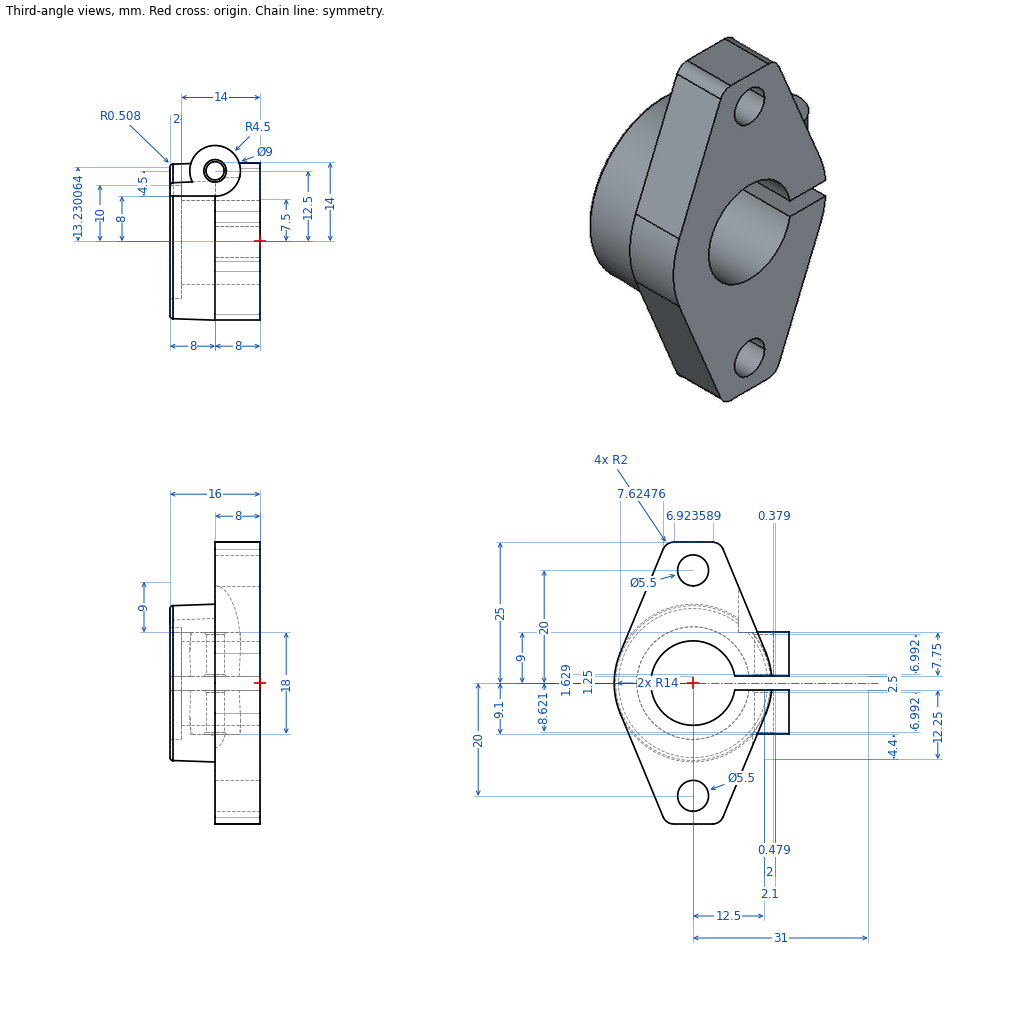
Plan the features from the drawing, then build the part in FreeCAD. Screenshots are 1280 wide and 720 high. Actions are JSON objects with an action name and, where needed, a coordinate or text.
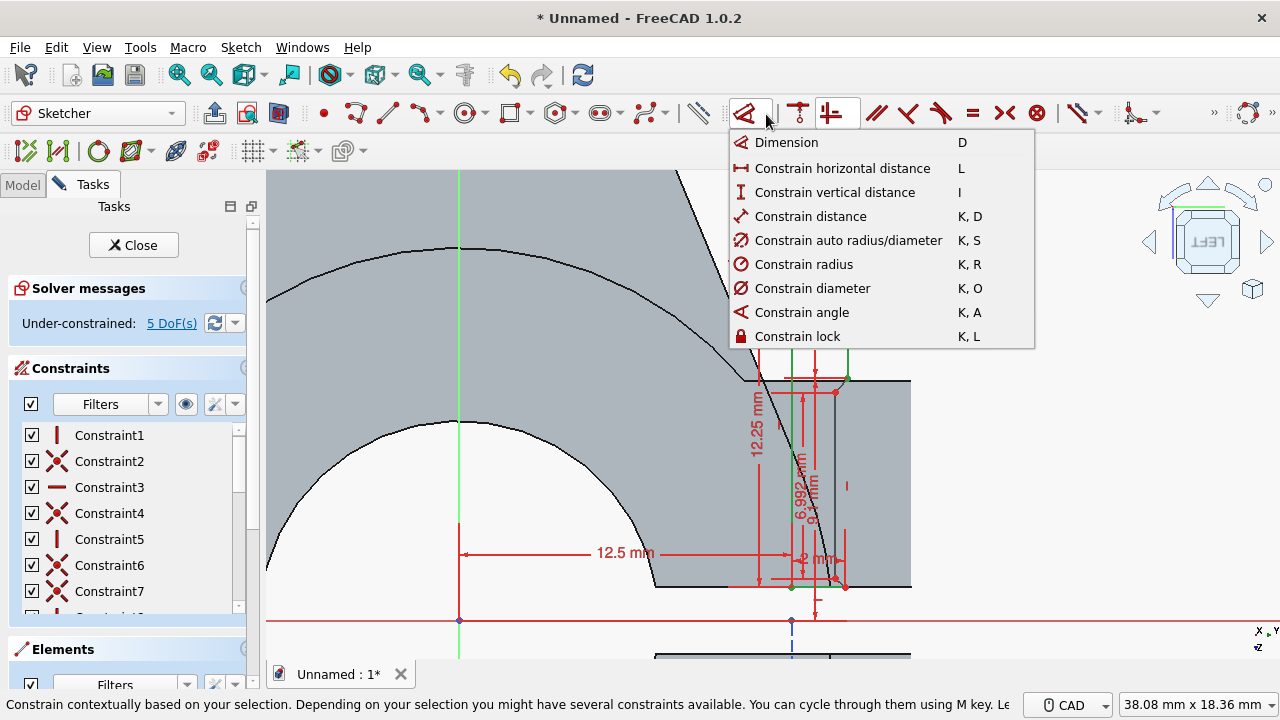
{"action": "left_click", "coordinate": [882, 168]}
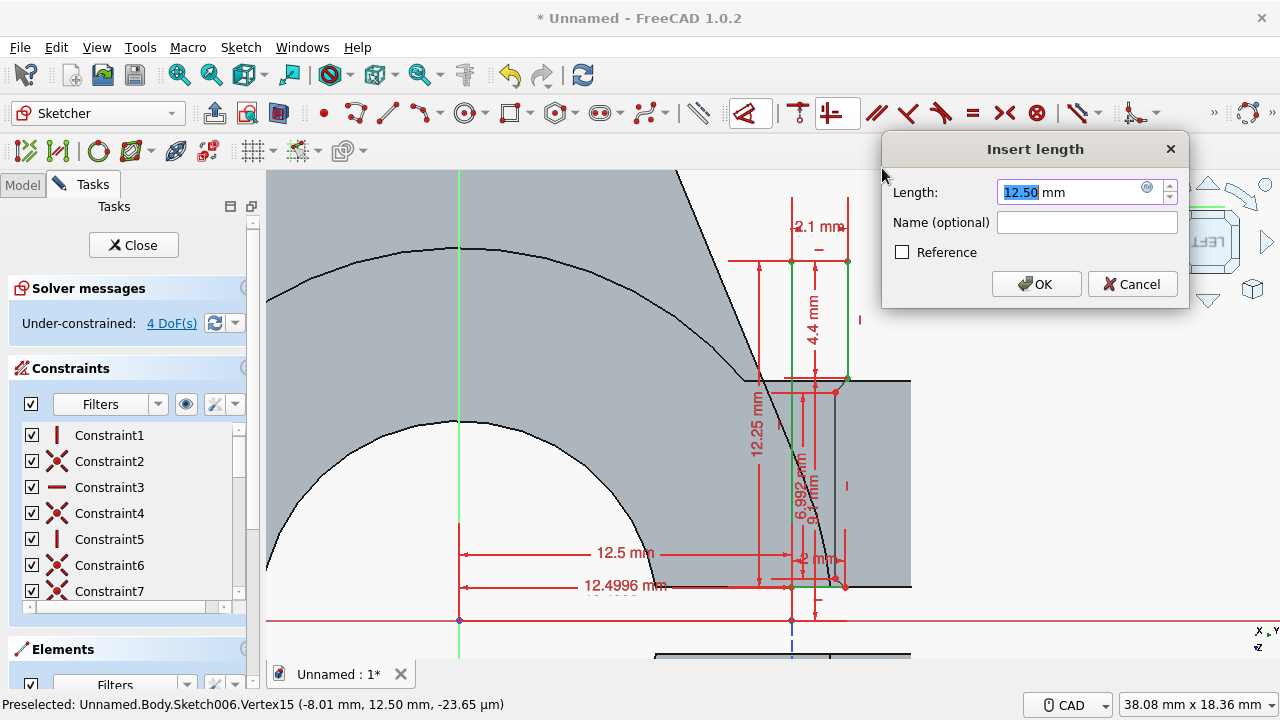
{"action": "type", "text": "12.5"}
{"action": "key", "text": "Return"}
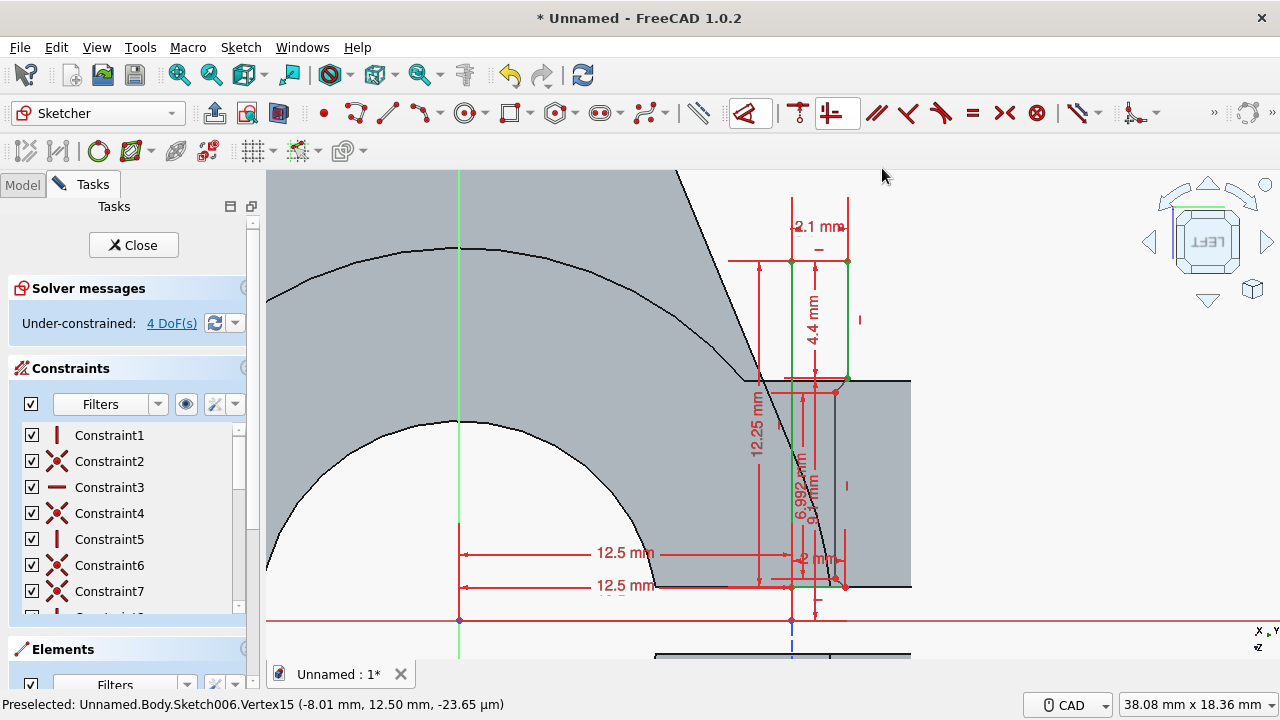
{"action": "left_click", "coordinate": [835, 393]}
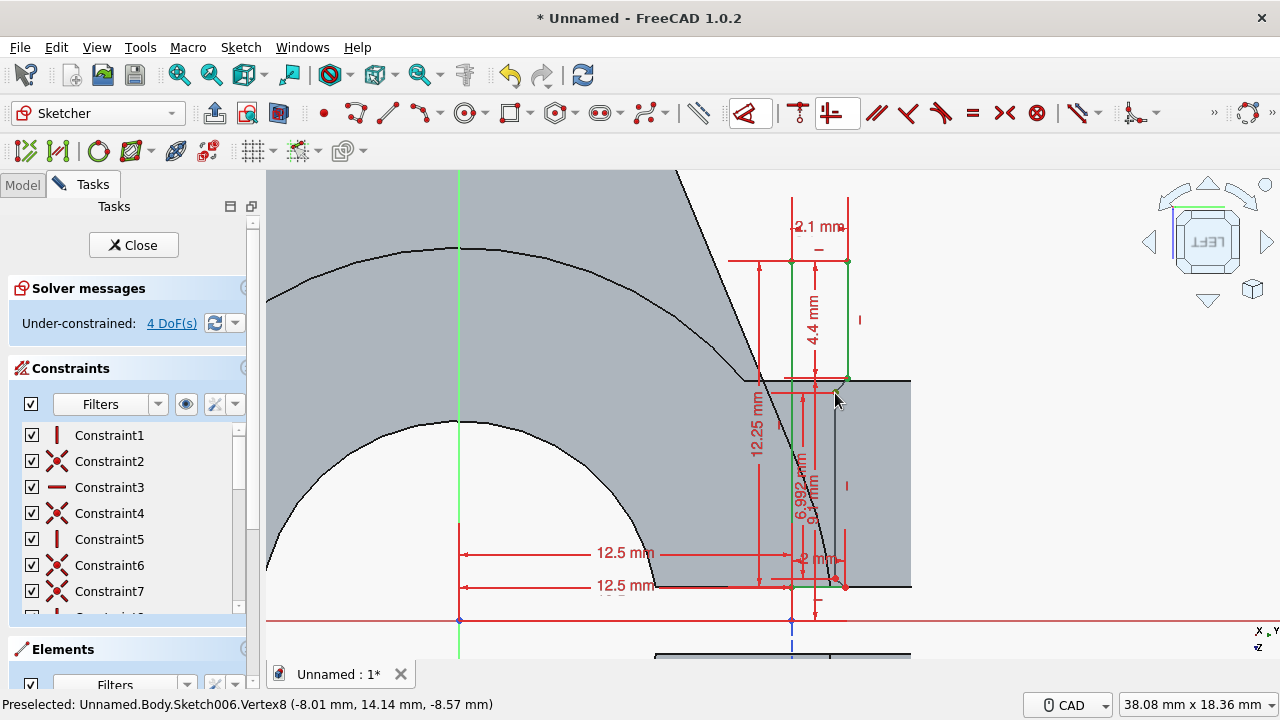
{"action": "left_click", "coordinate": [766, 114]}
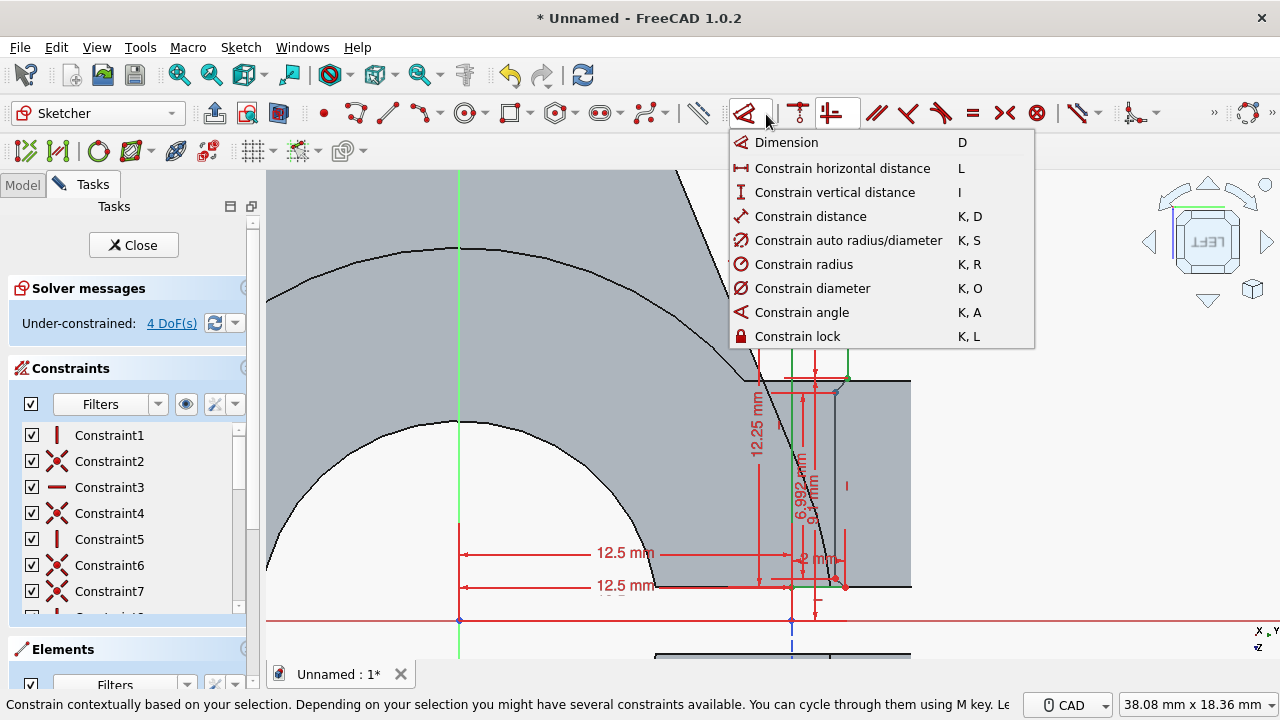
{"action": "left_click", "coordinate": [882, 192]}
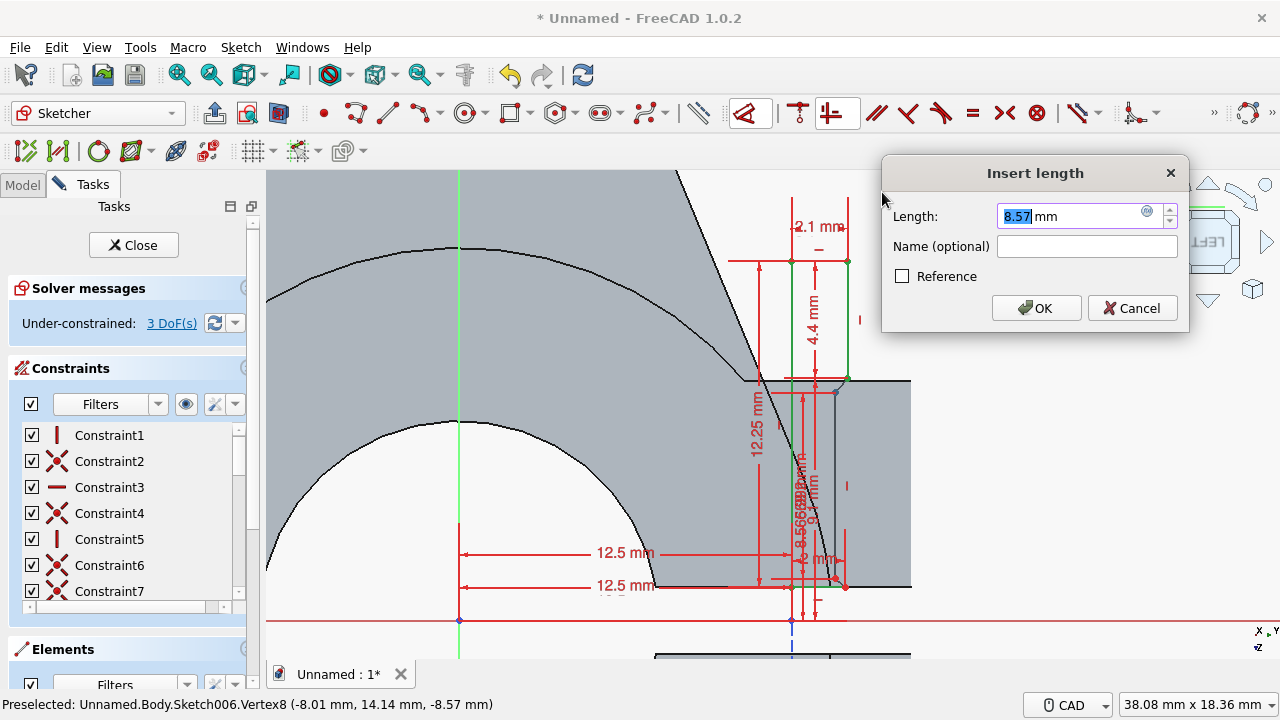
{"action": "type", "text": "8.621"}
{"action": "key", "text": "Return"}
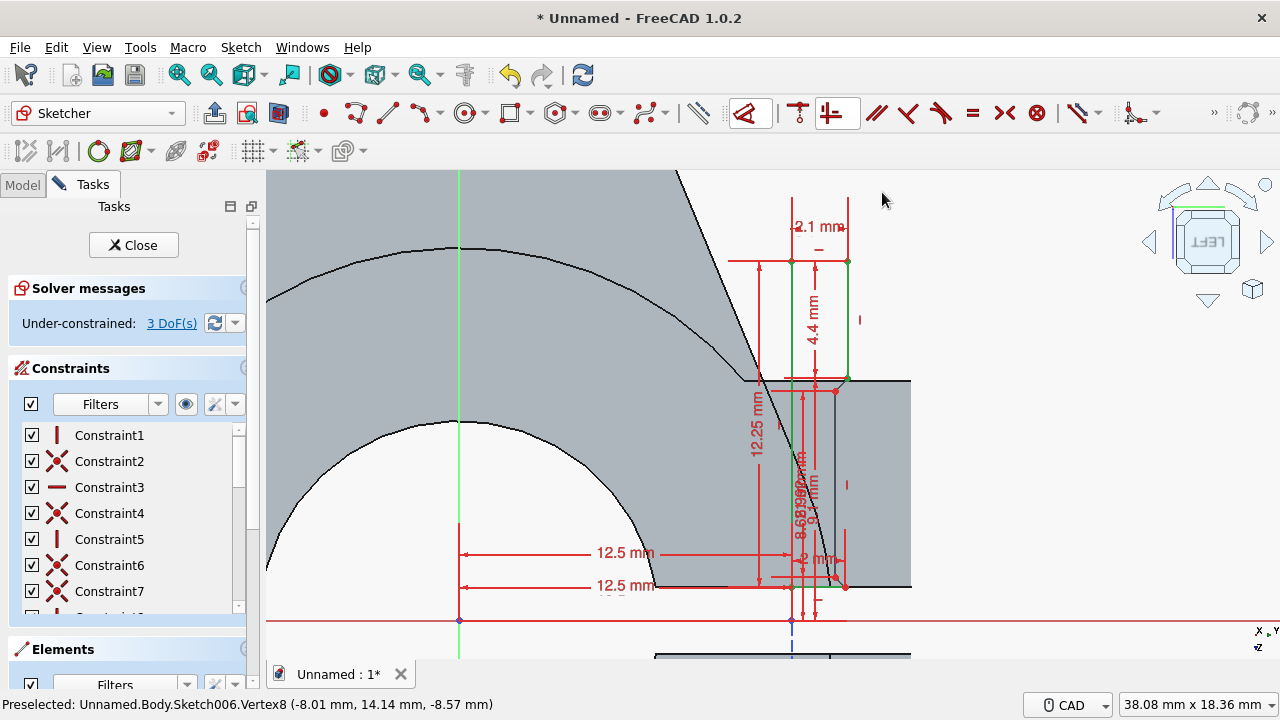
{"action": "scroll", "coordinate": [842, 385], "scroll_direction": "up", "scroll_amount": 6}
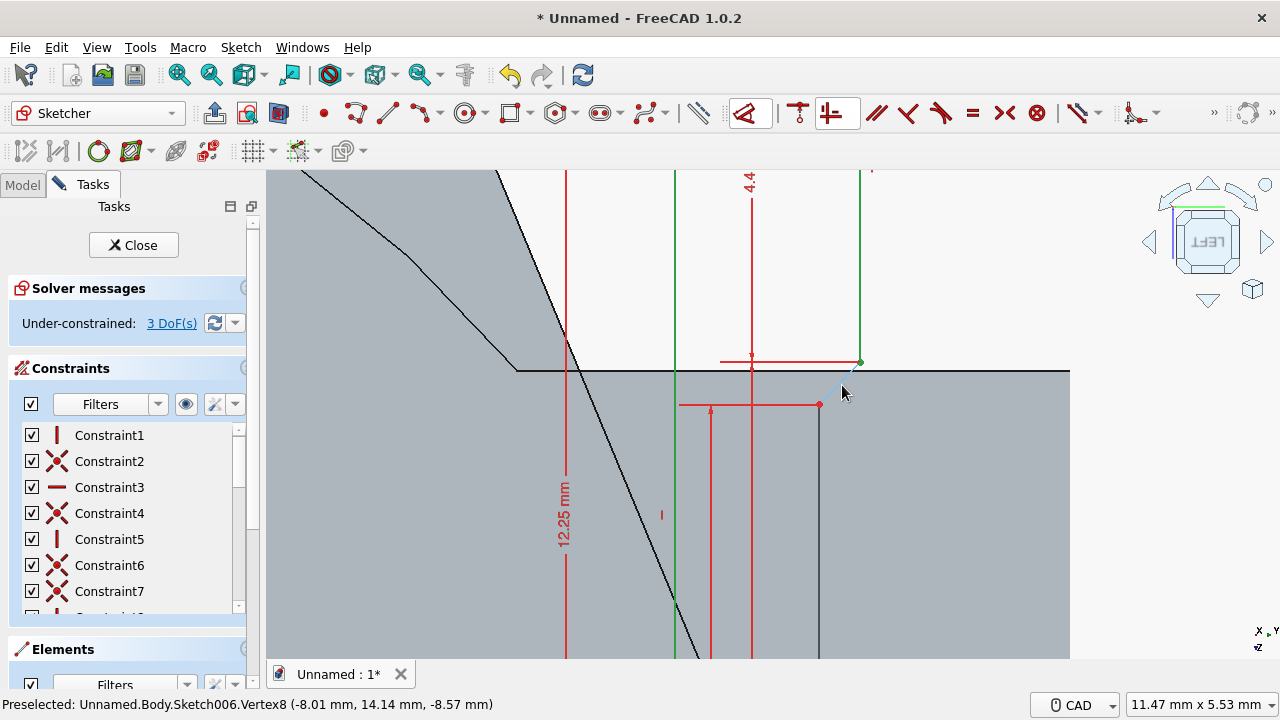
{"action": "left_click", "coordinate": [840, 383]}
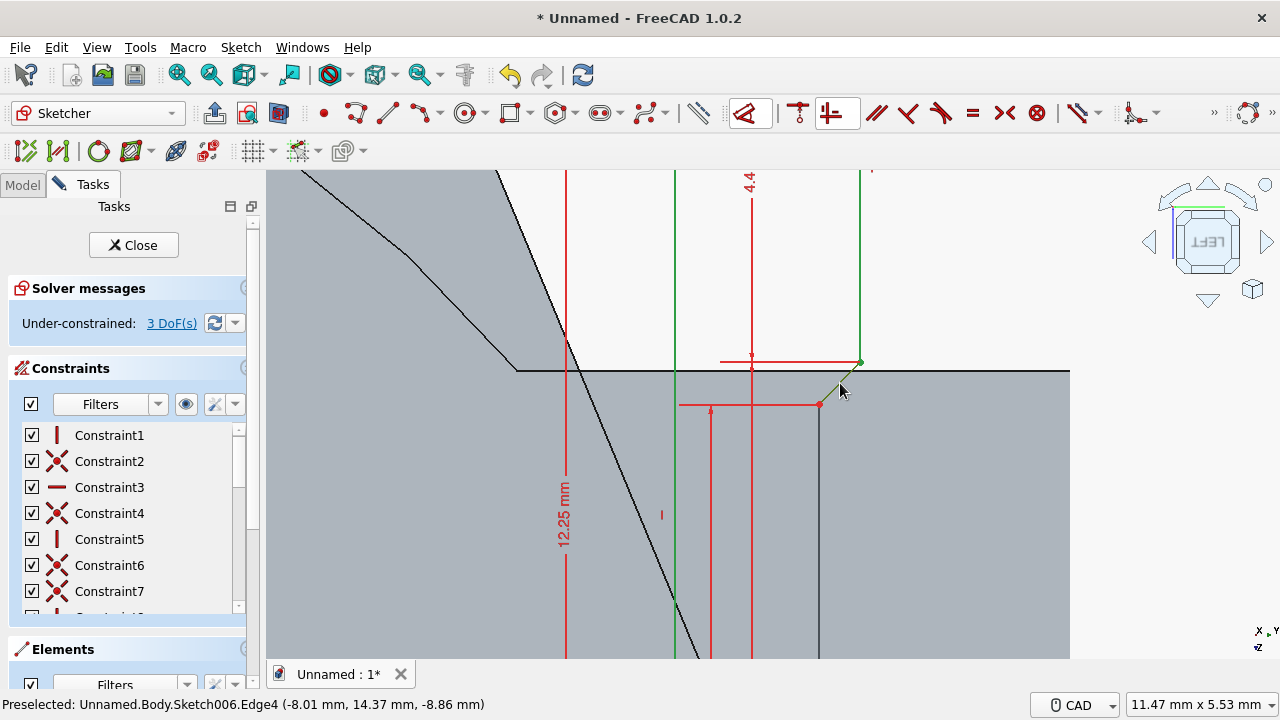
{"action": "key", "text": "l"}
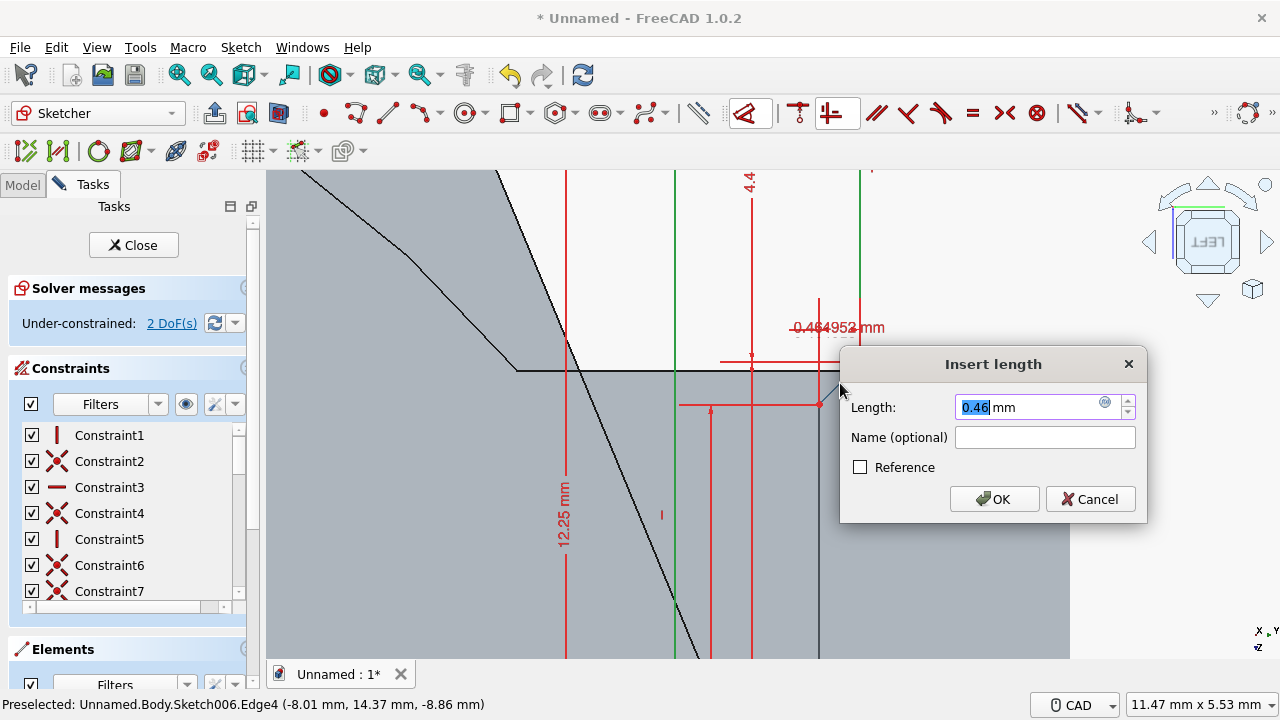
{"action": "type", "text": "0.479"}
{"action": "key", "text": "Return"}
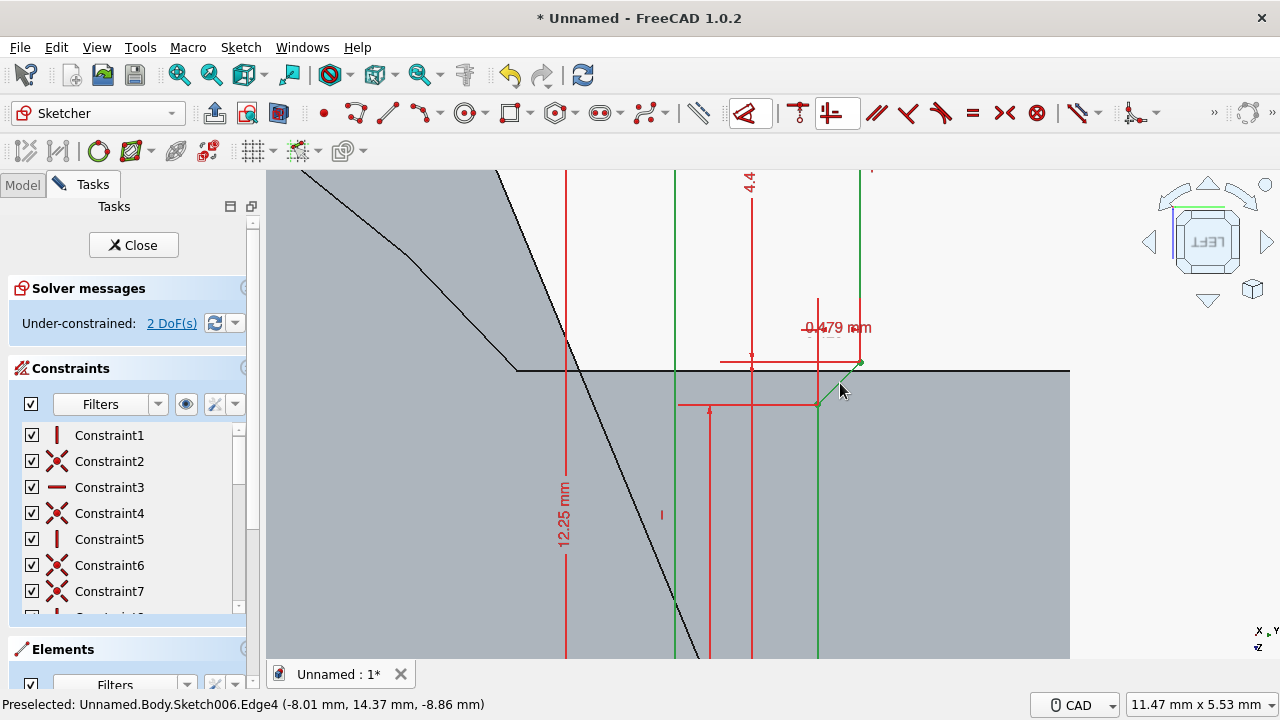
{"action": "left_click", "coordinate": [134, 245]}